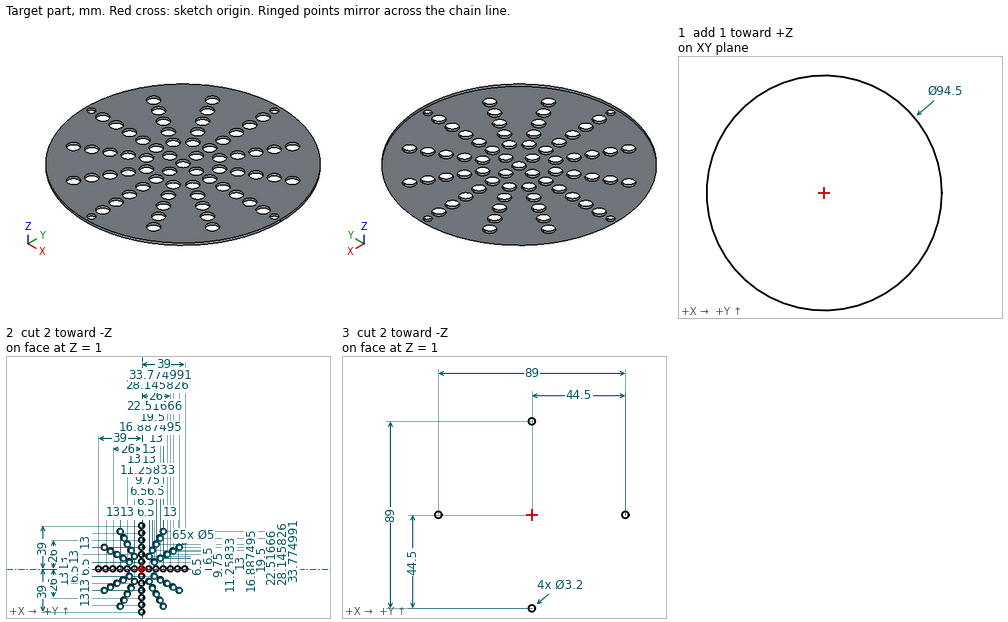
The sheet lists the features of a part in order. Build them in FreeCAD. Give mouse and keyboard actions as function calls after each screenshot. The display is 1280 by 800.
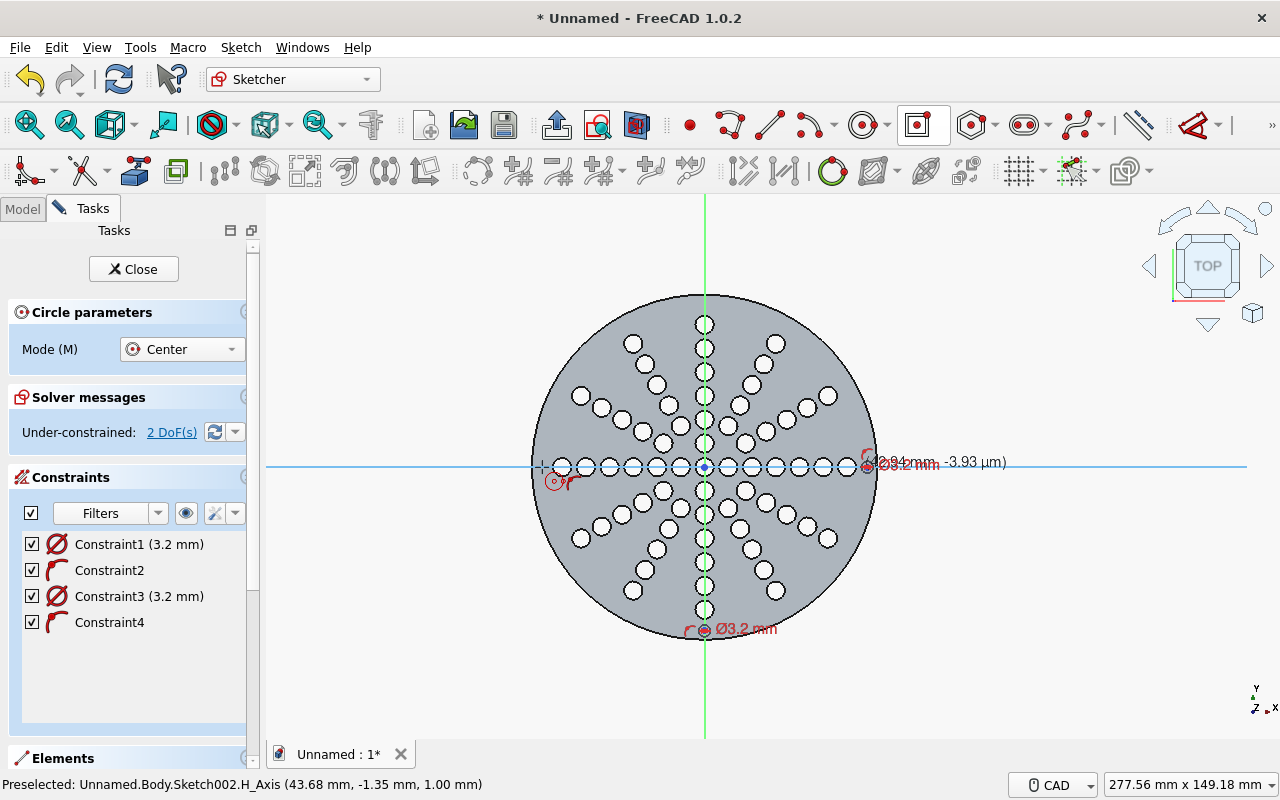
click(542, 467)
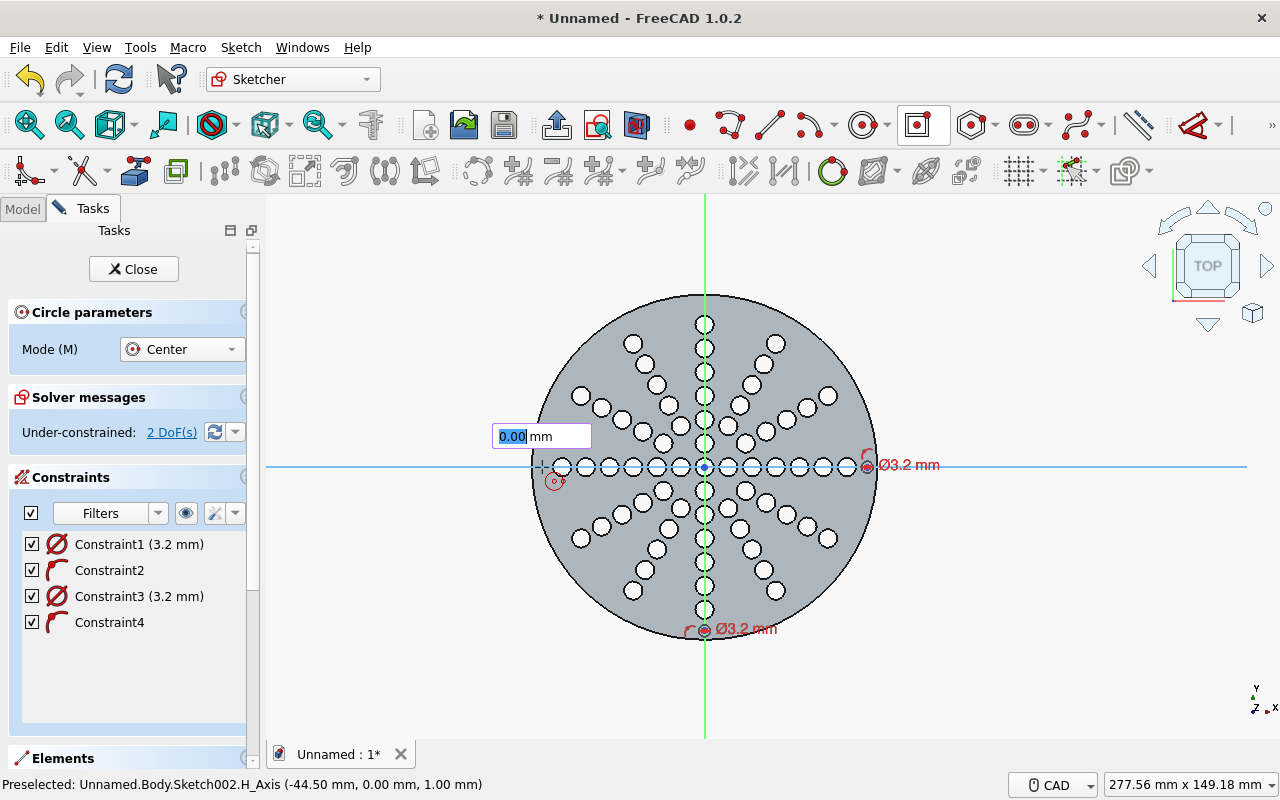
scroll(540, 473, up, 6)
move(539, 471)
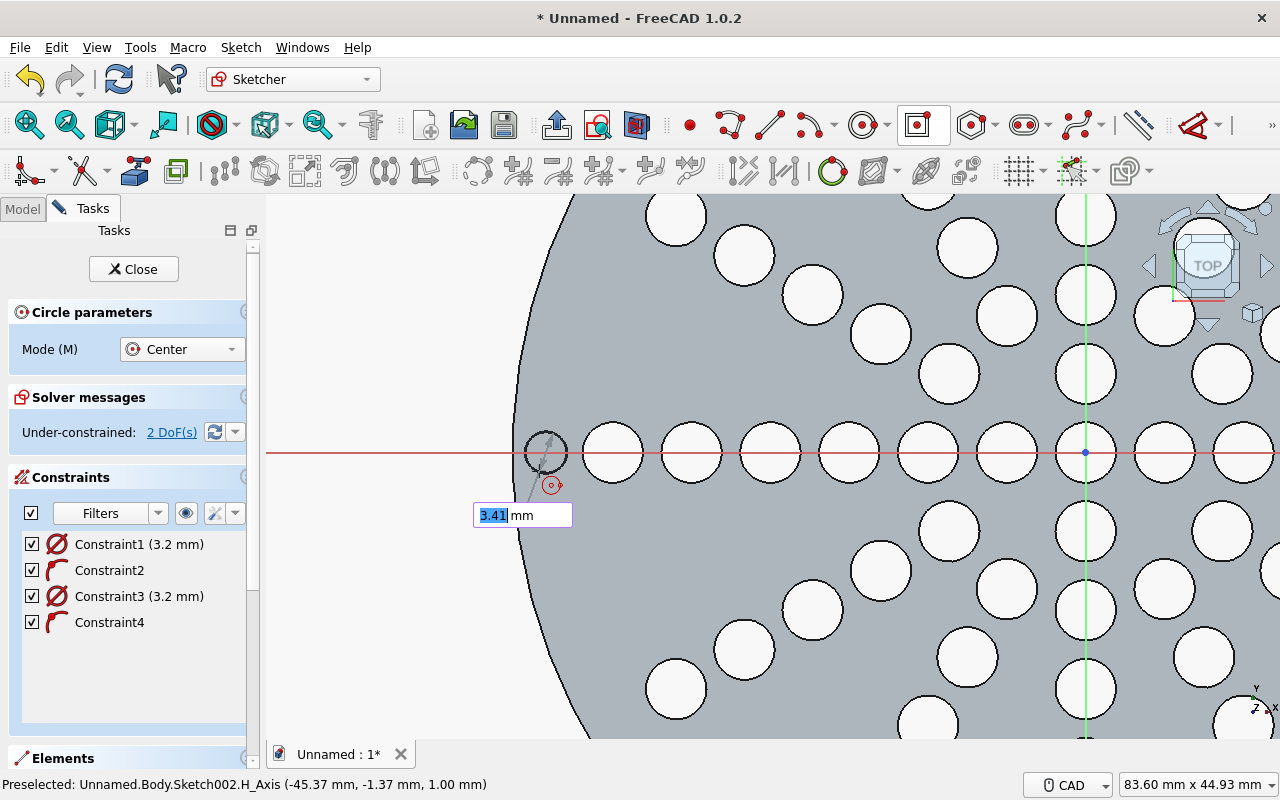
text(3.2)
key(Return)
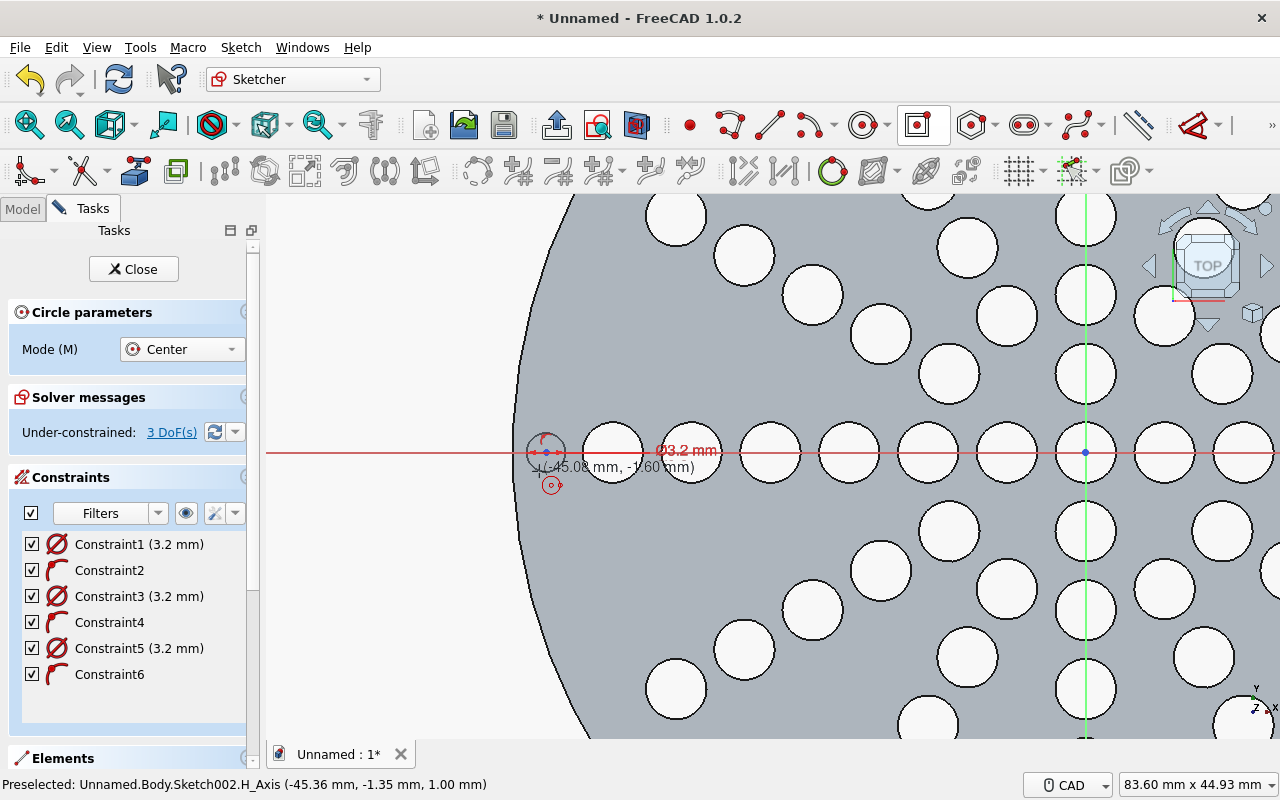
scroll(540, 473, down, 6)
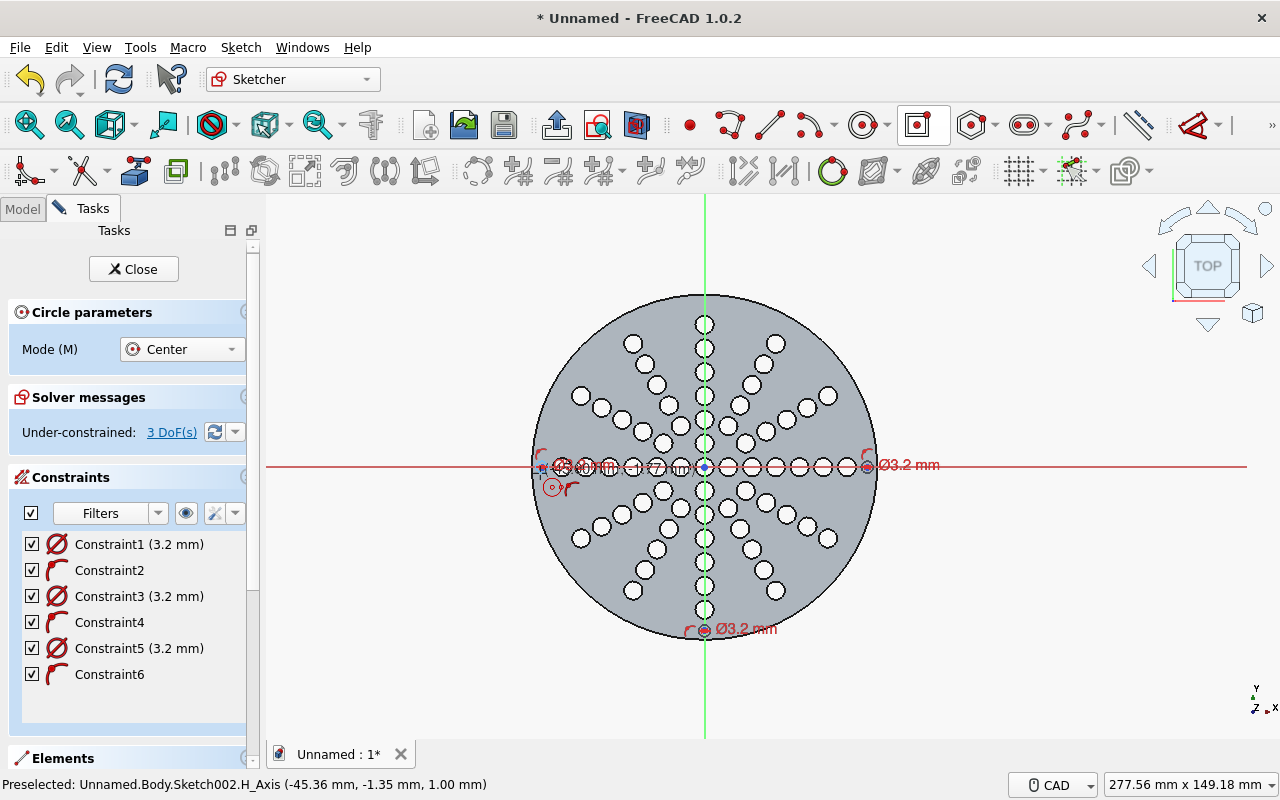
scroll(705, 305, up, 7)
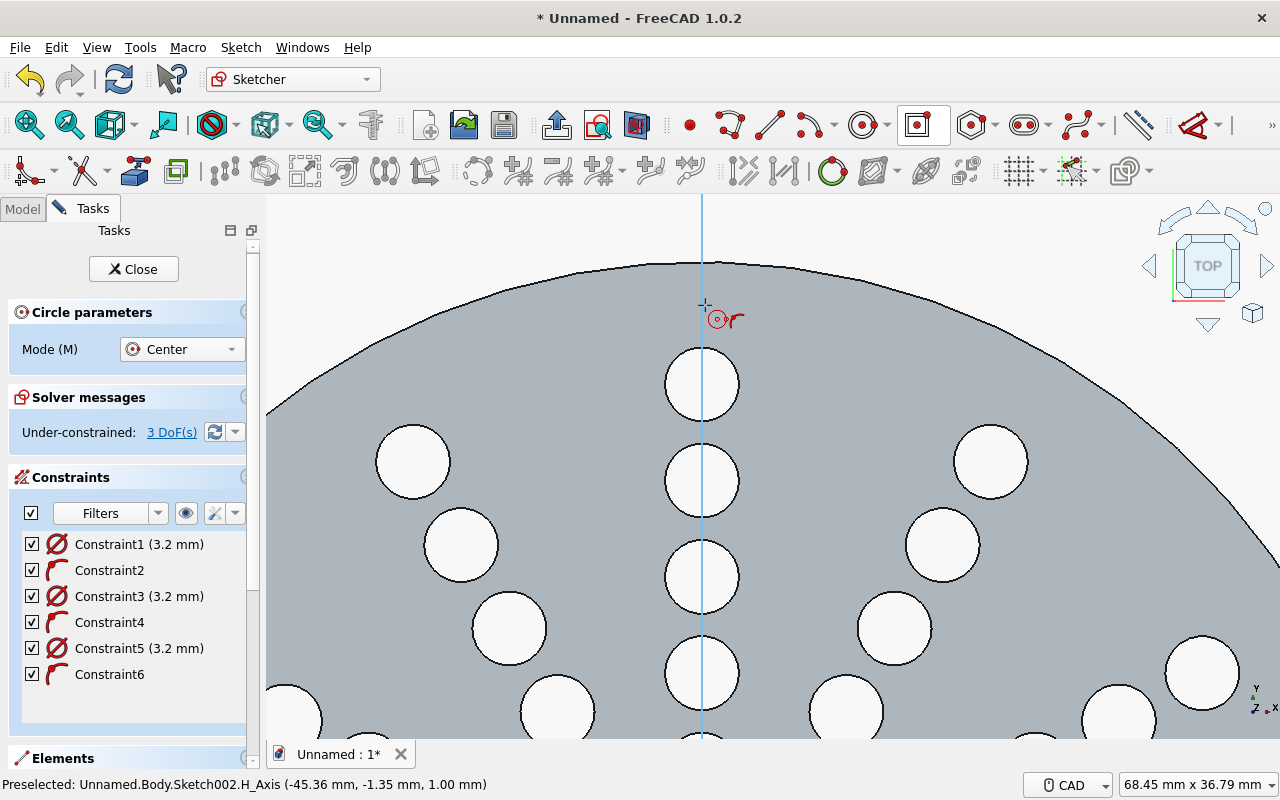
scroll(705, 304, down, 7)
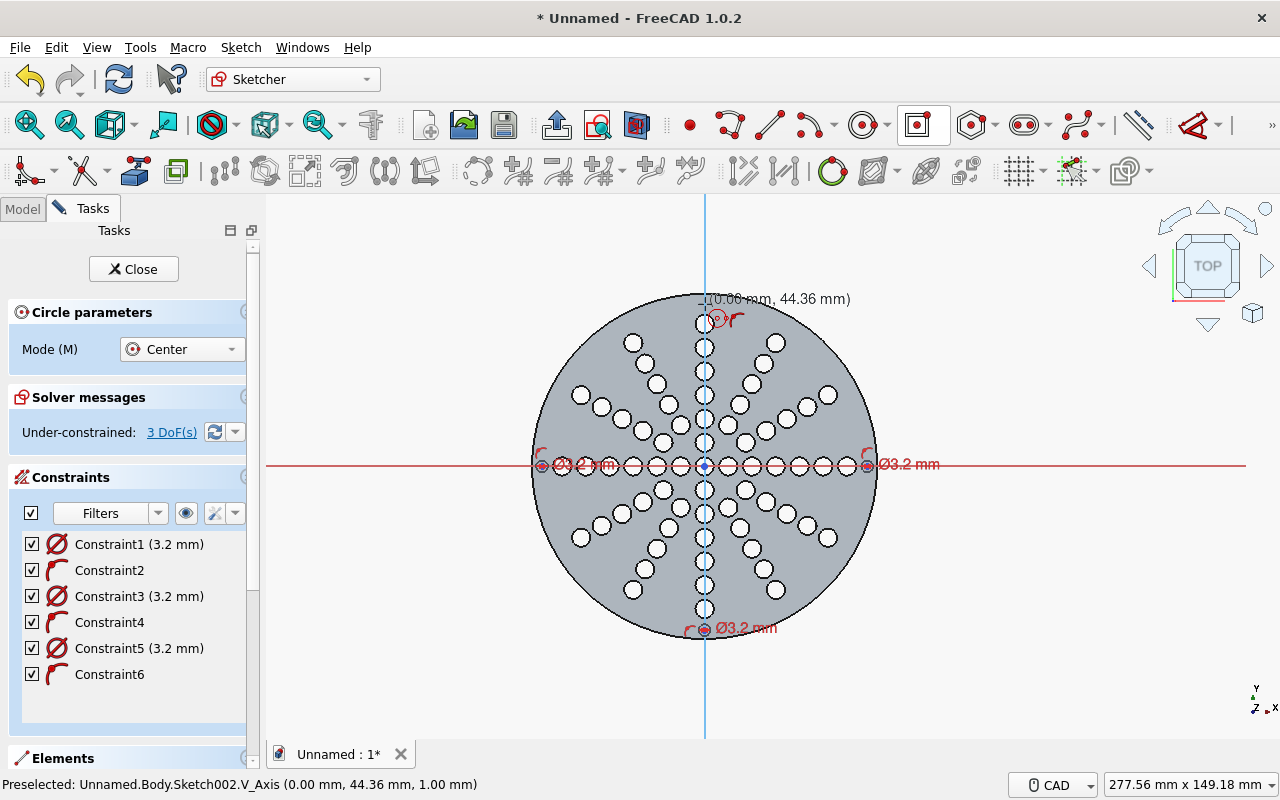
click(705, 304)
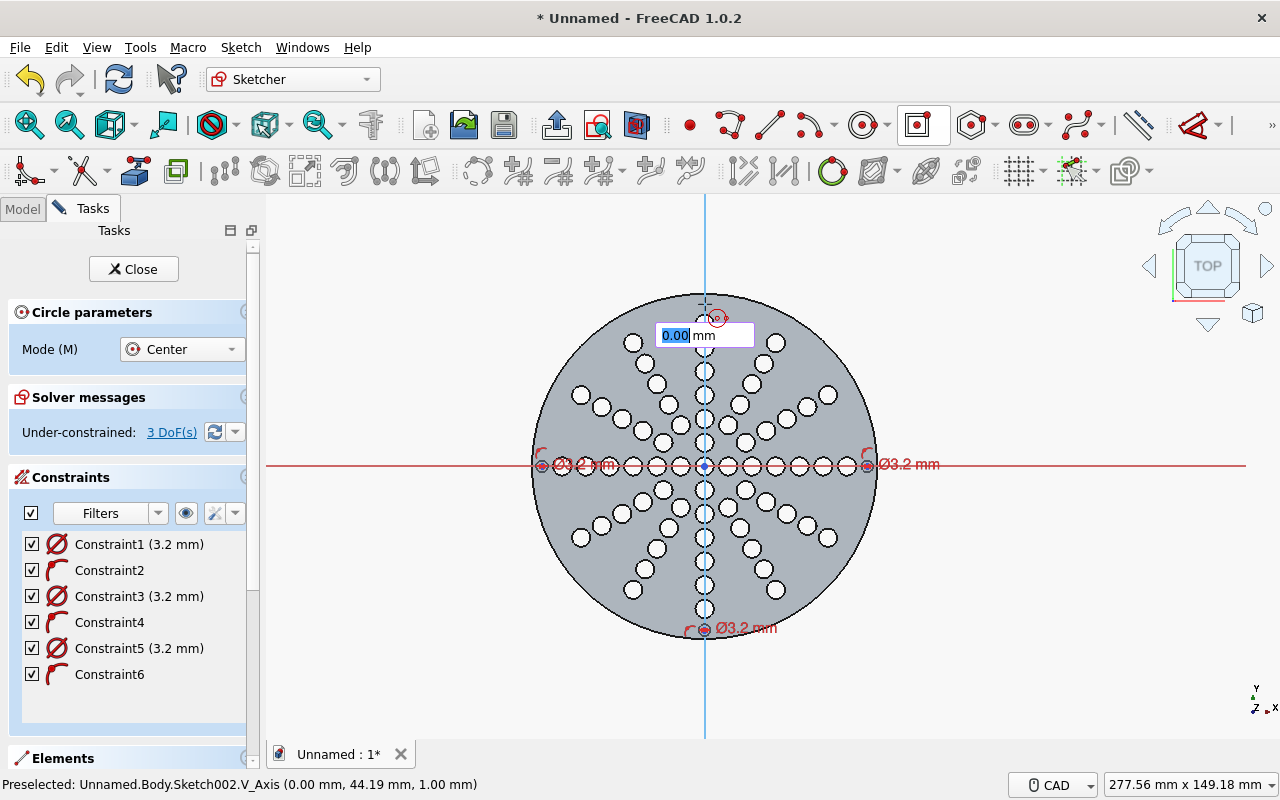
scroll(710, 302, up, 6)
move(709, 301)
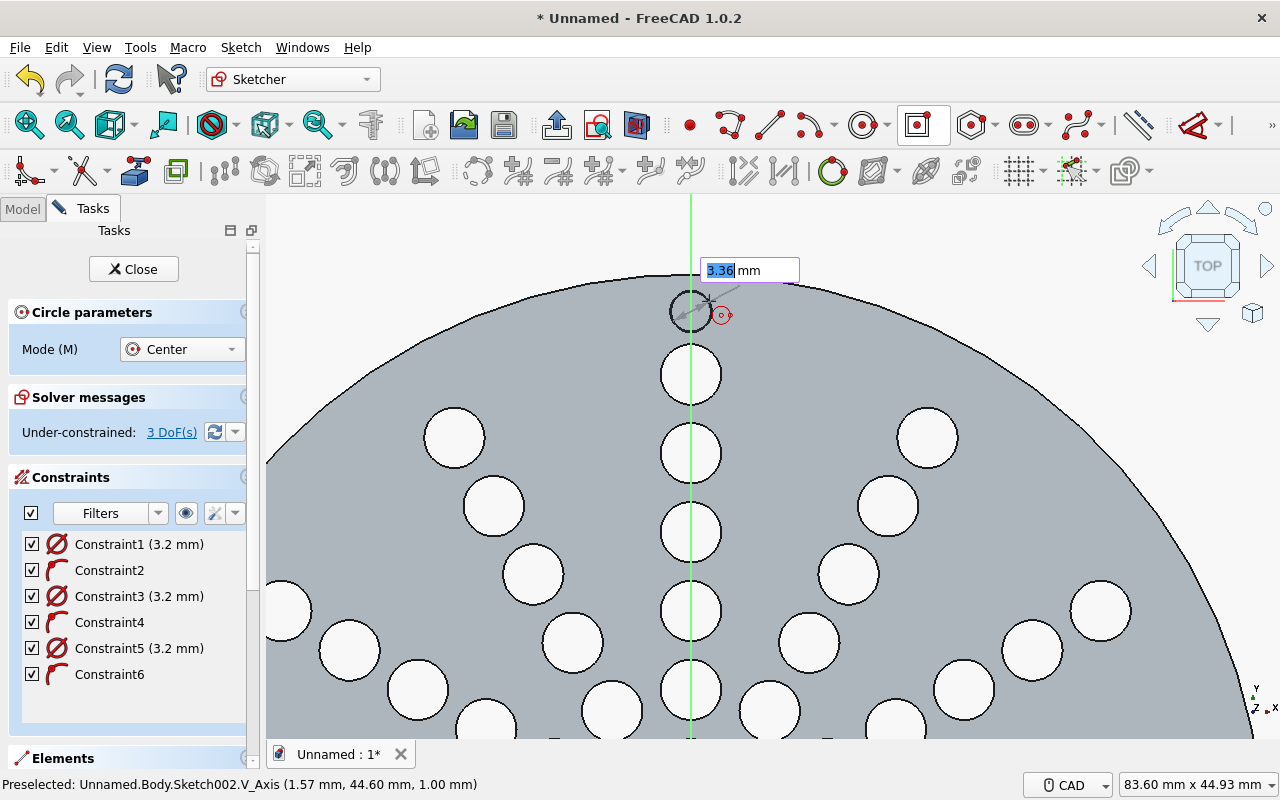
text(3.2)
key(Return)
key(Escape)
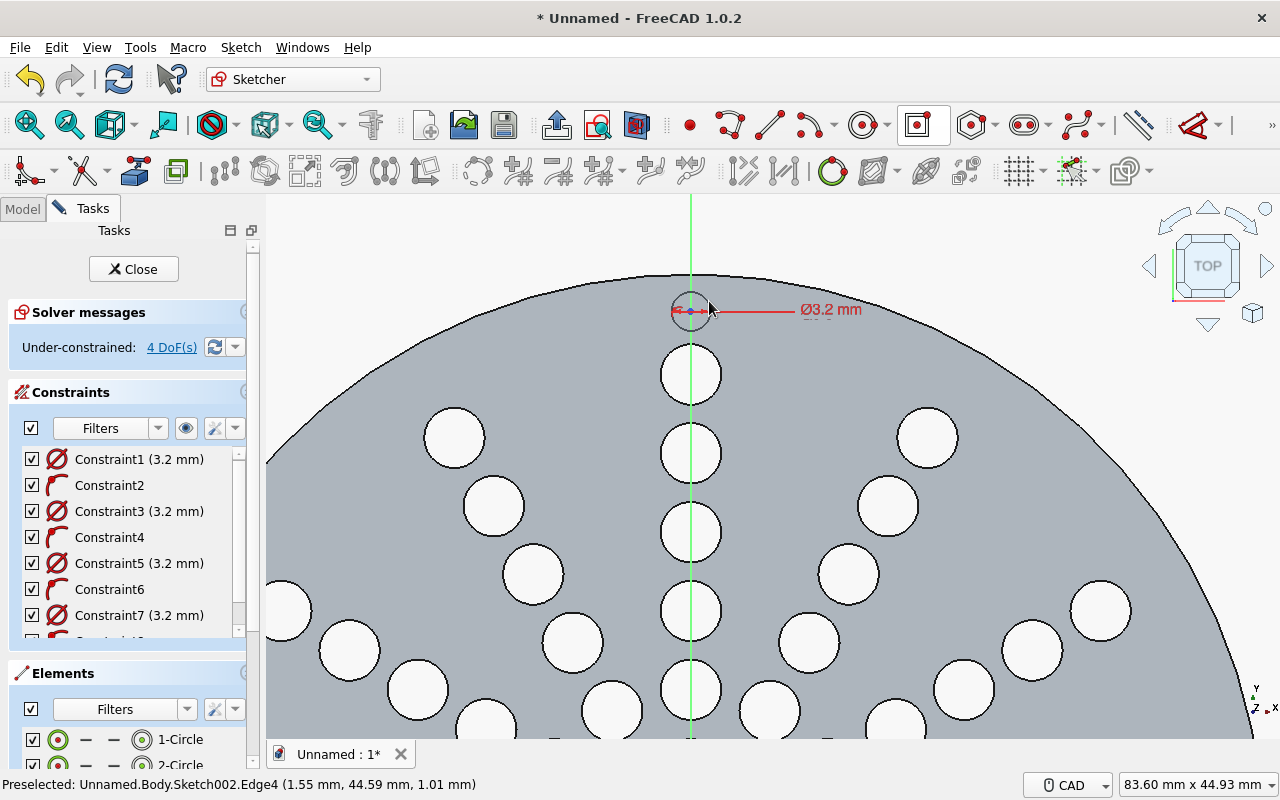
key(d)